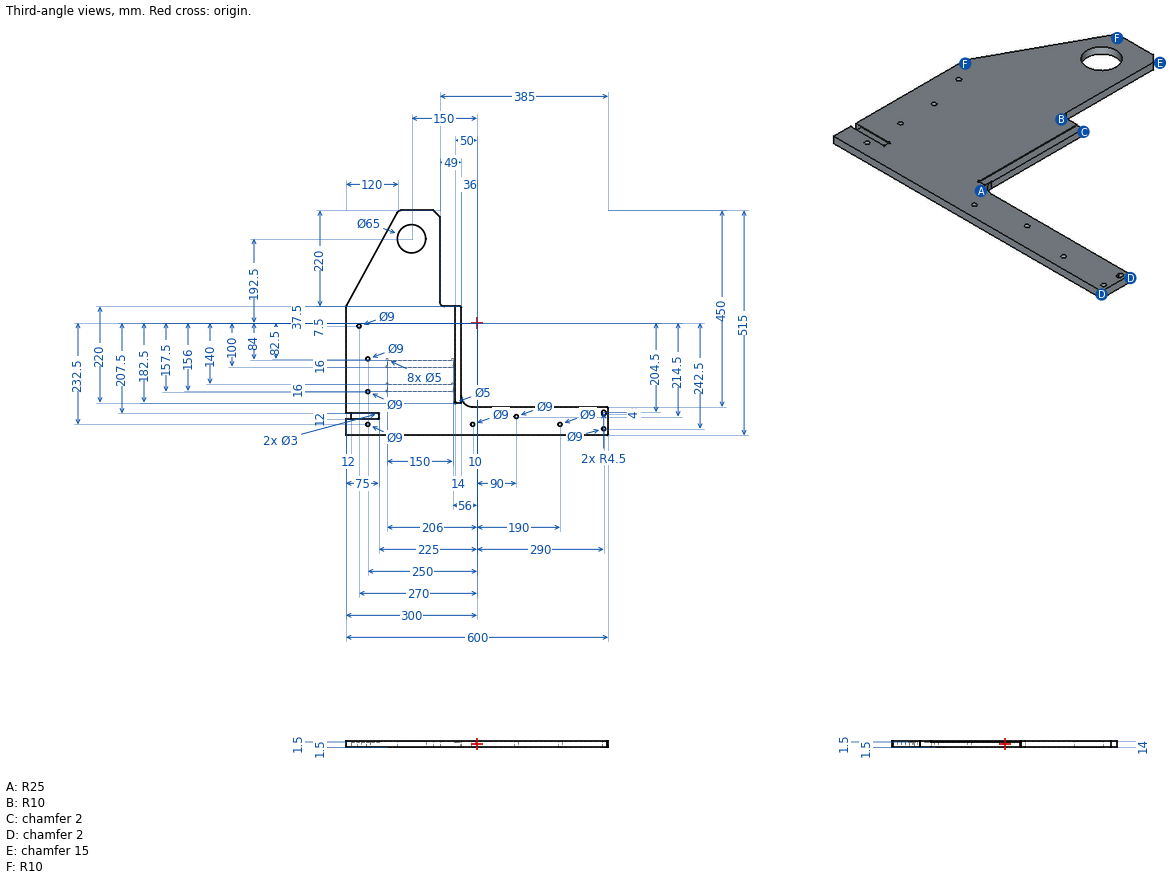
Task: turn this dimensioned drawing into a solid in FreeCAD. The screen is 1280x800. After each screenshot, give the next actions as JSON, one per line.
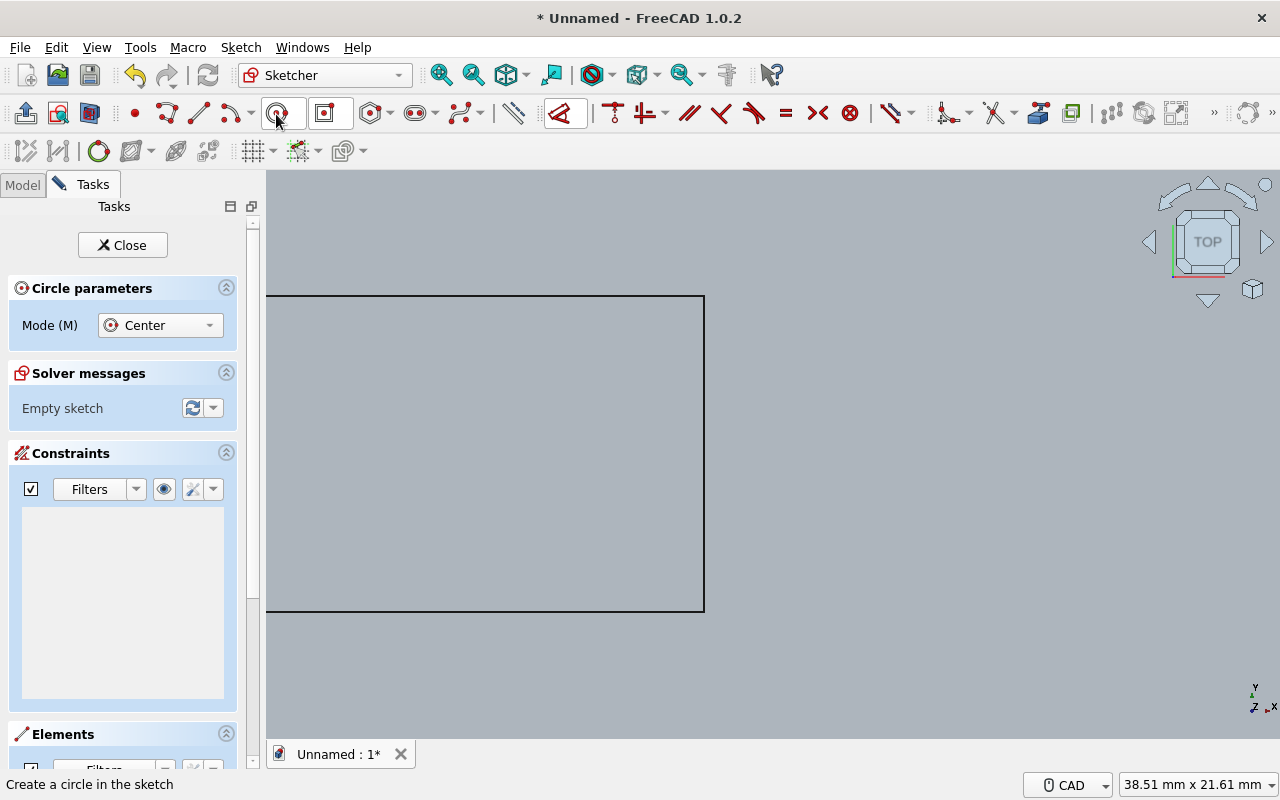
{"action": "left_click", "coordinate": [704, 296]}
{"action": "mouse_move", "coordinate": [732, 268]}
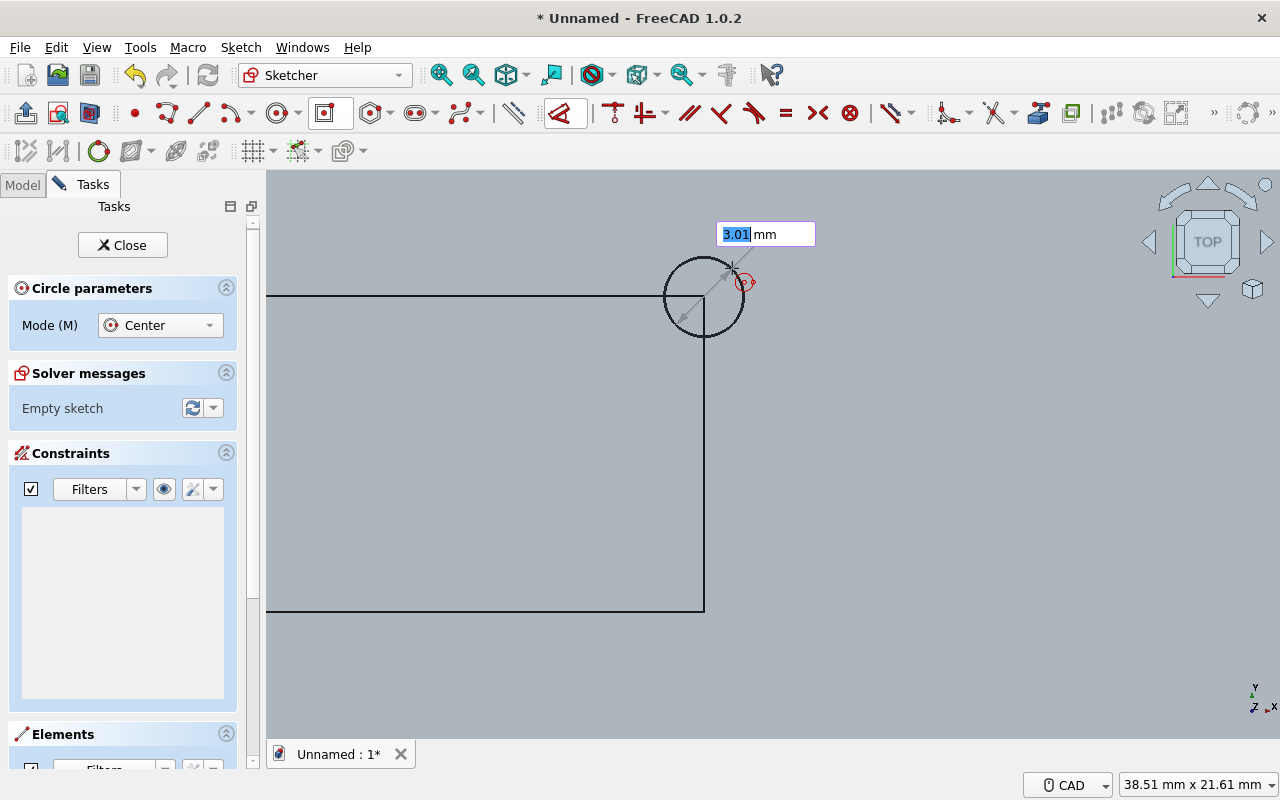
{"action": "type", "text": "3"}
{"action": "key", "text": "Return"}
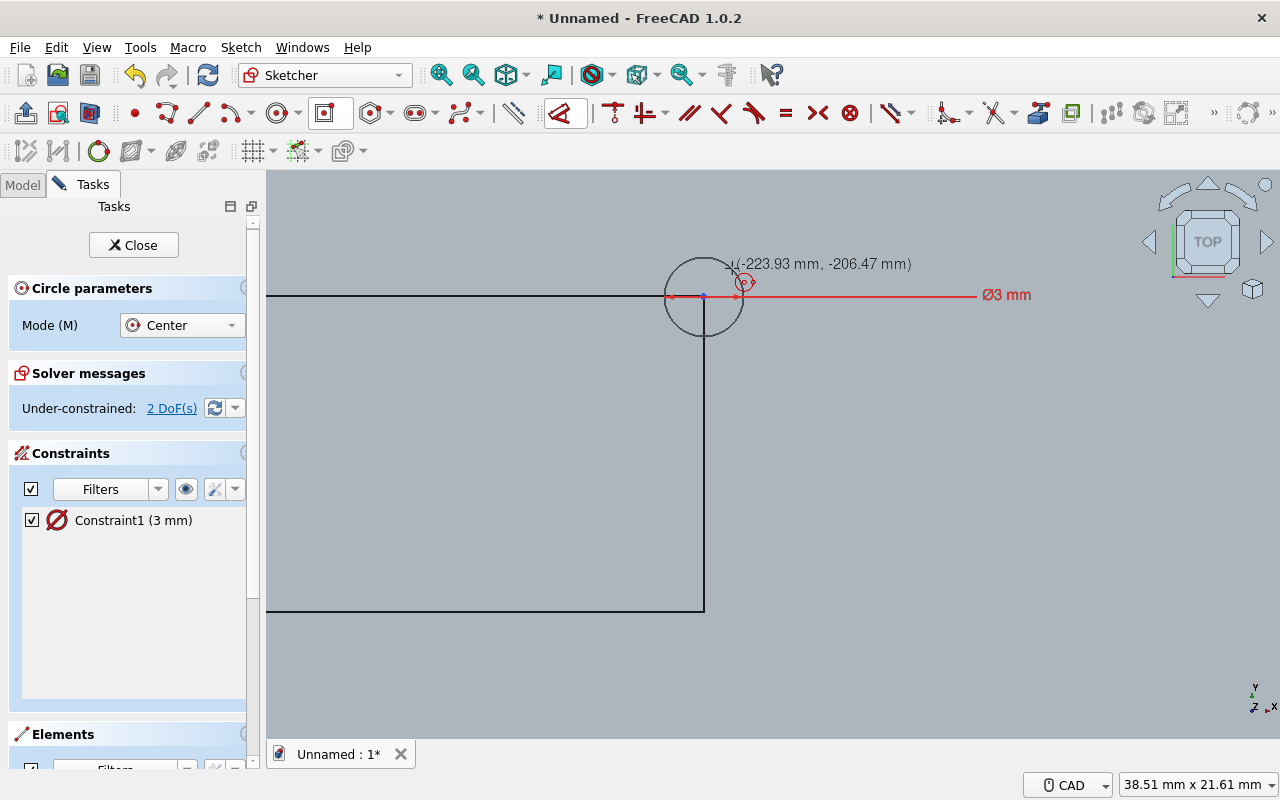
{"action": "left_click", "coordinate": [704, 612]}
{"action": "mouse_move", "coordinate": [732, 584]}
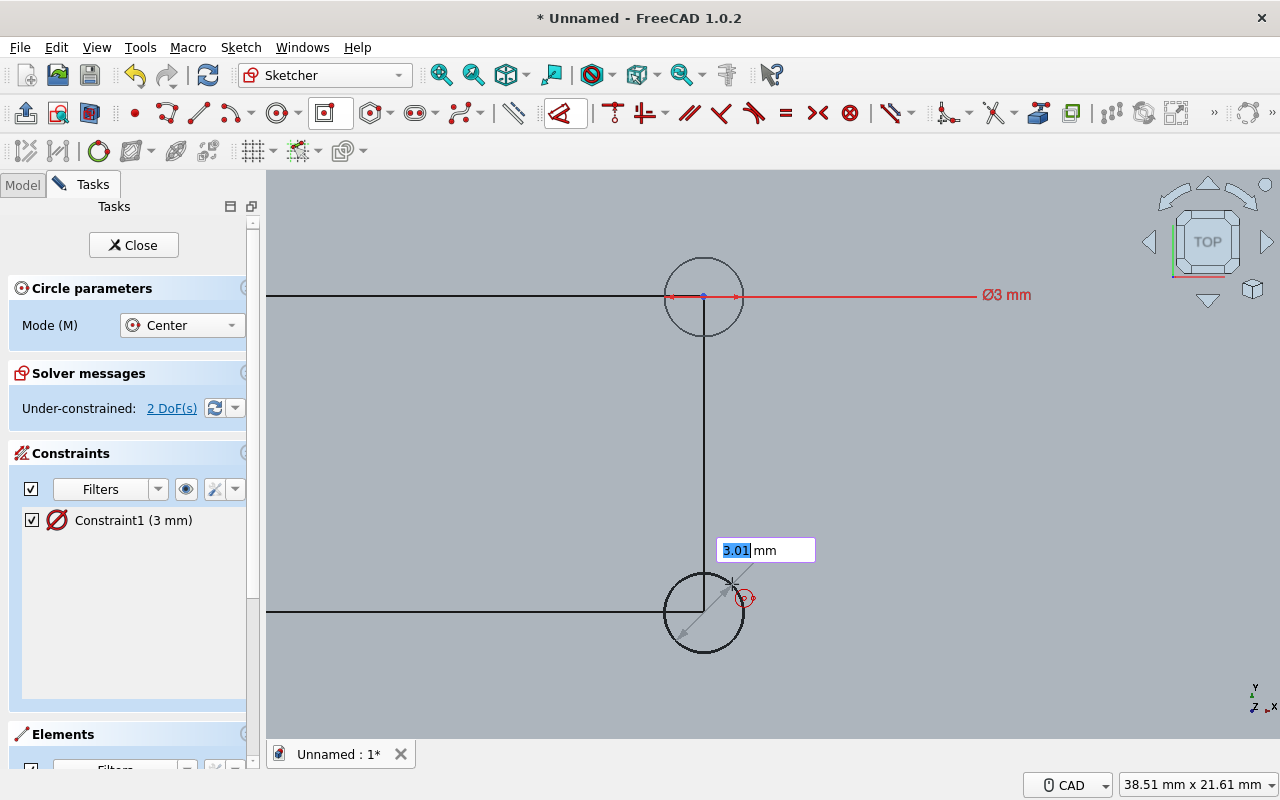
{"action": "type", "text": "3"}
{"action": "key", "text": "Return"}
{"action": "key", "text": "Escape"}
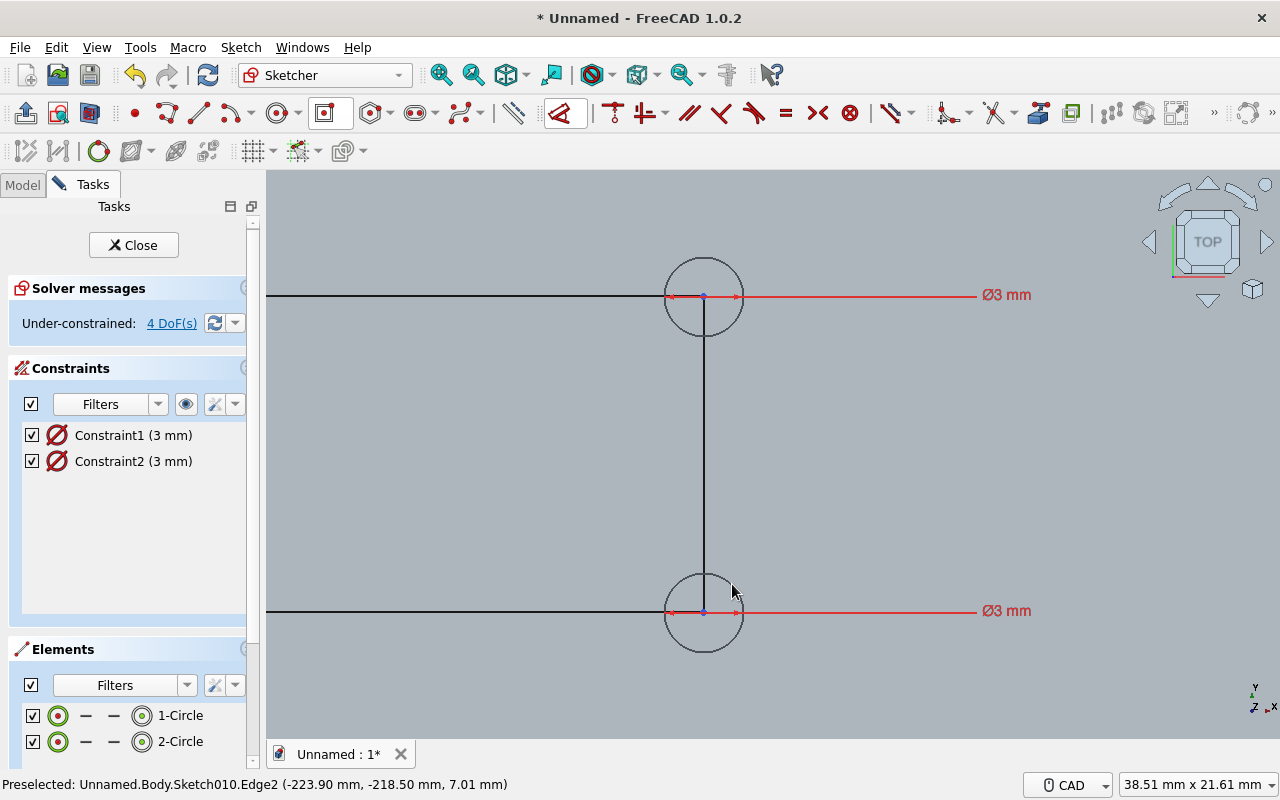
{"action": "left_click", "coordinate": [704, 297]}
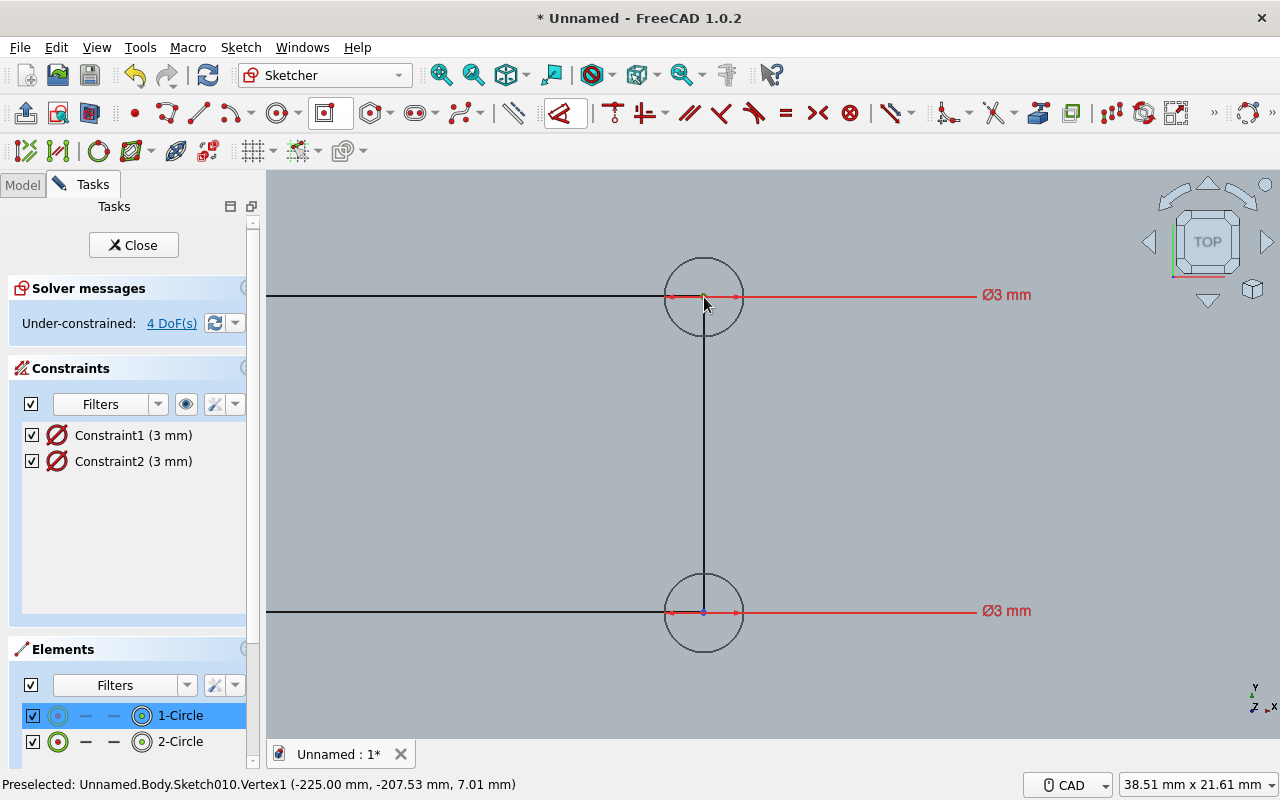
{"action": "key", "text": "l"}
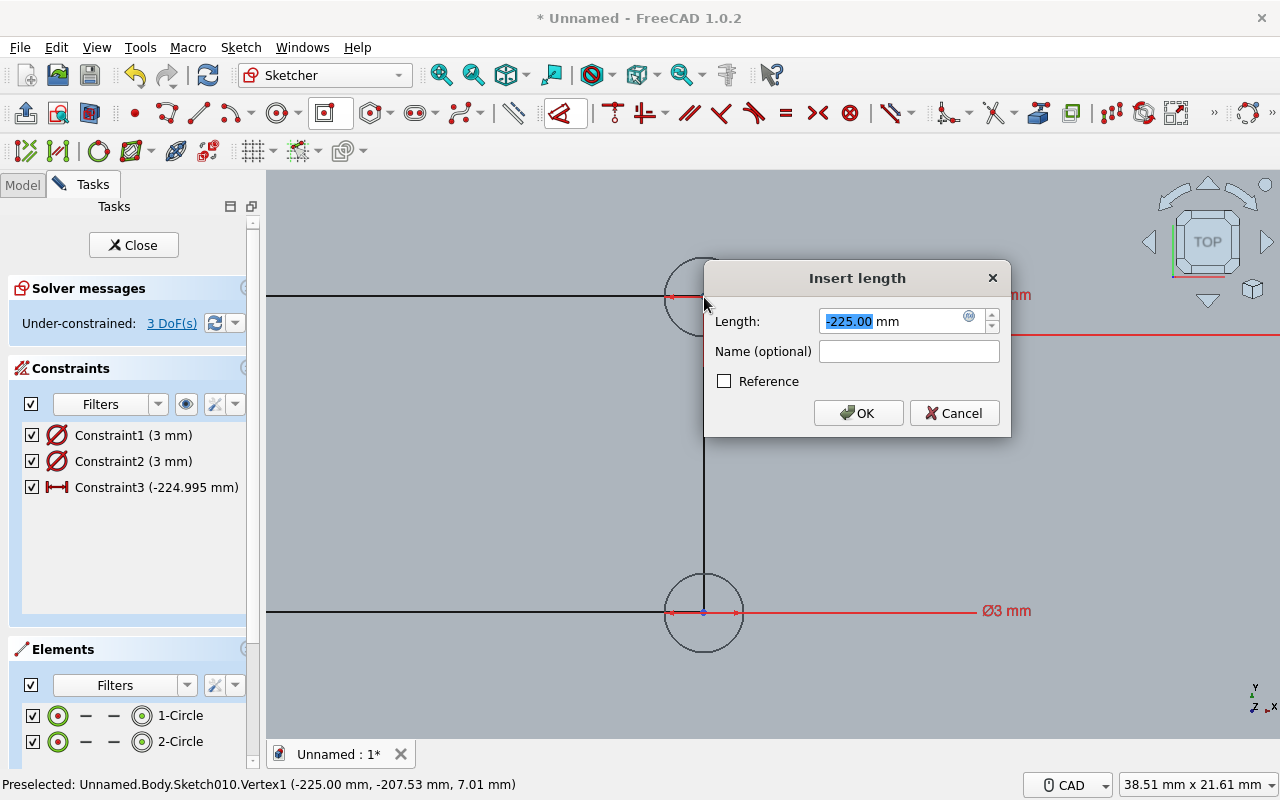
{"action": "type", "text": "-225"}
{"action": "key", "text": "Return"}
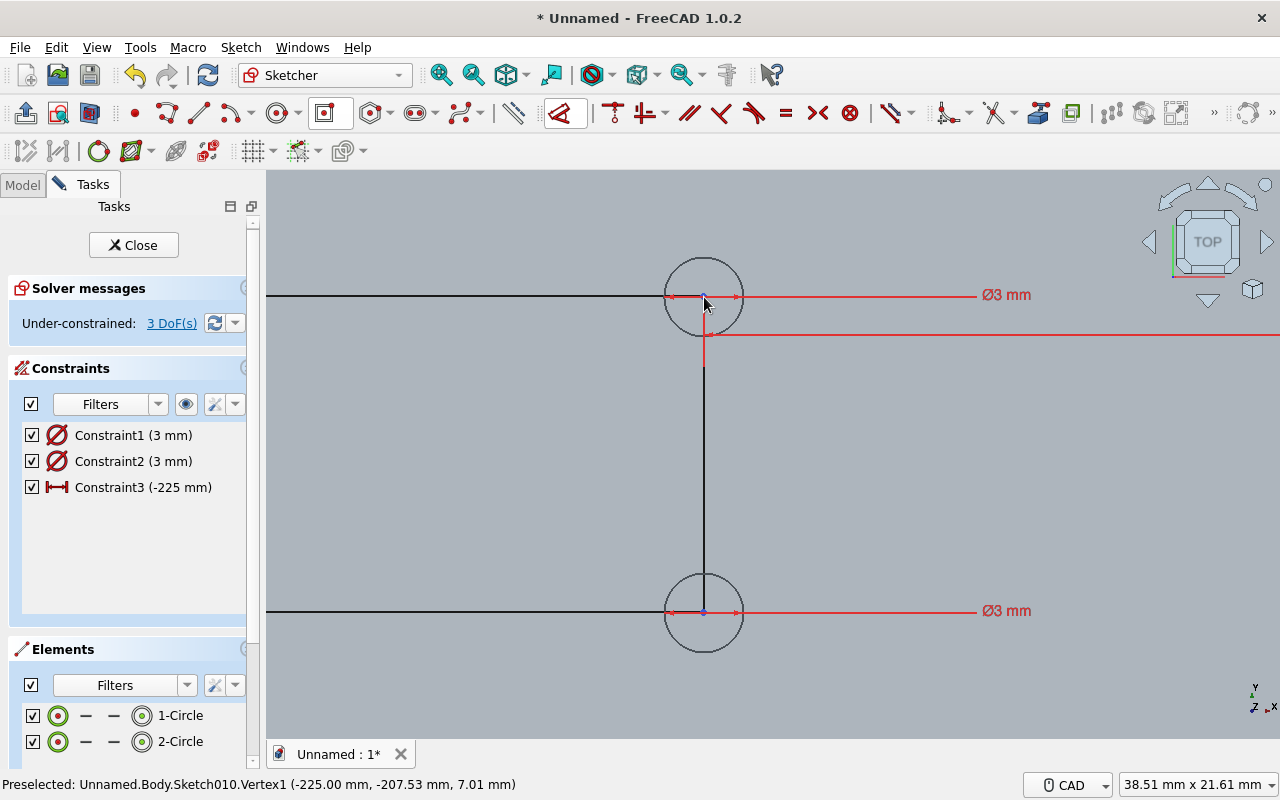
{"action": "left_click", "coordinate": [704, 613]}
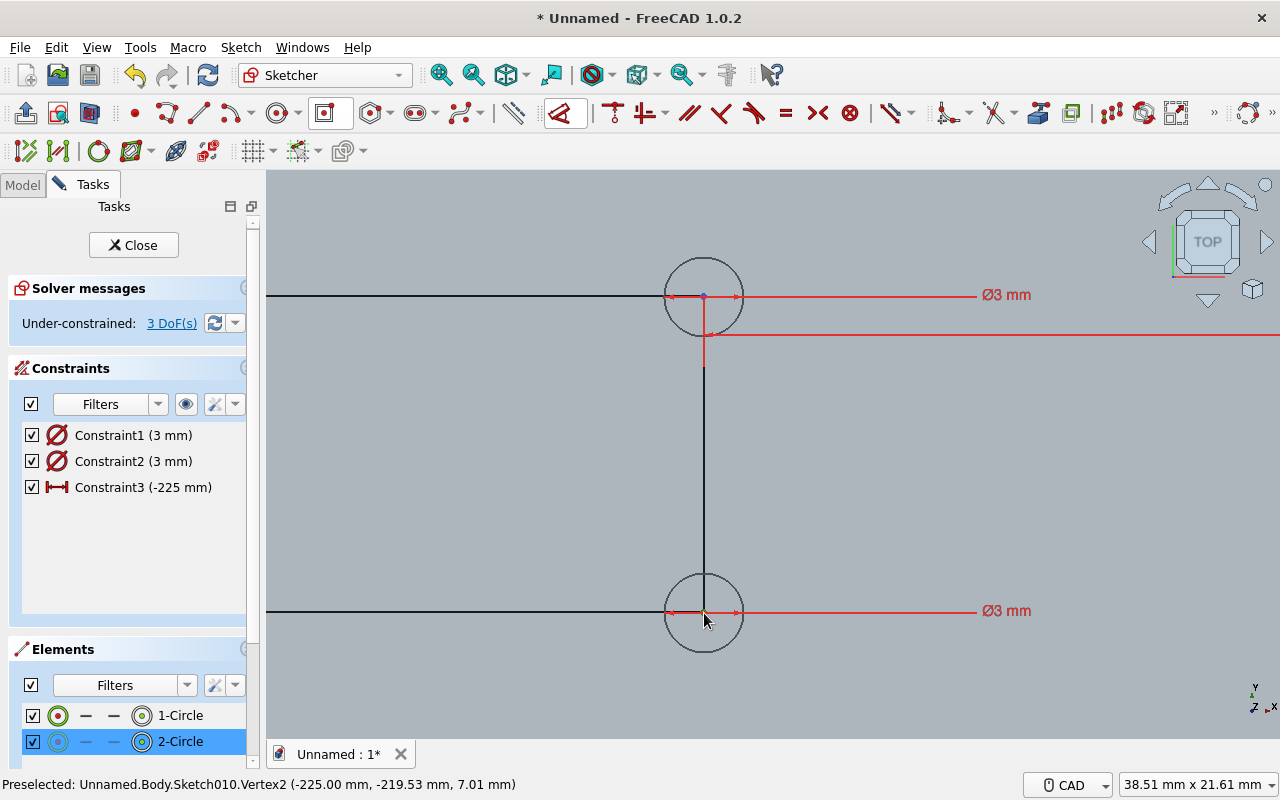
{"action": "left_click", "coordinate": [582, 114]}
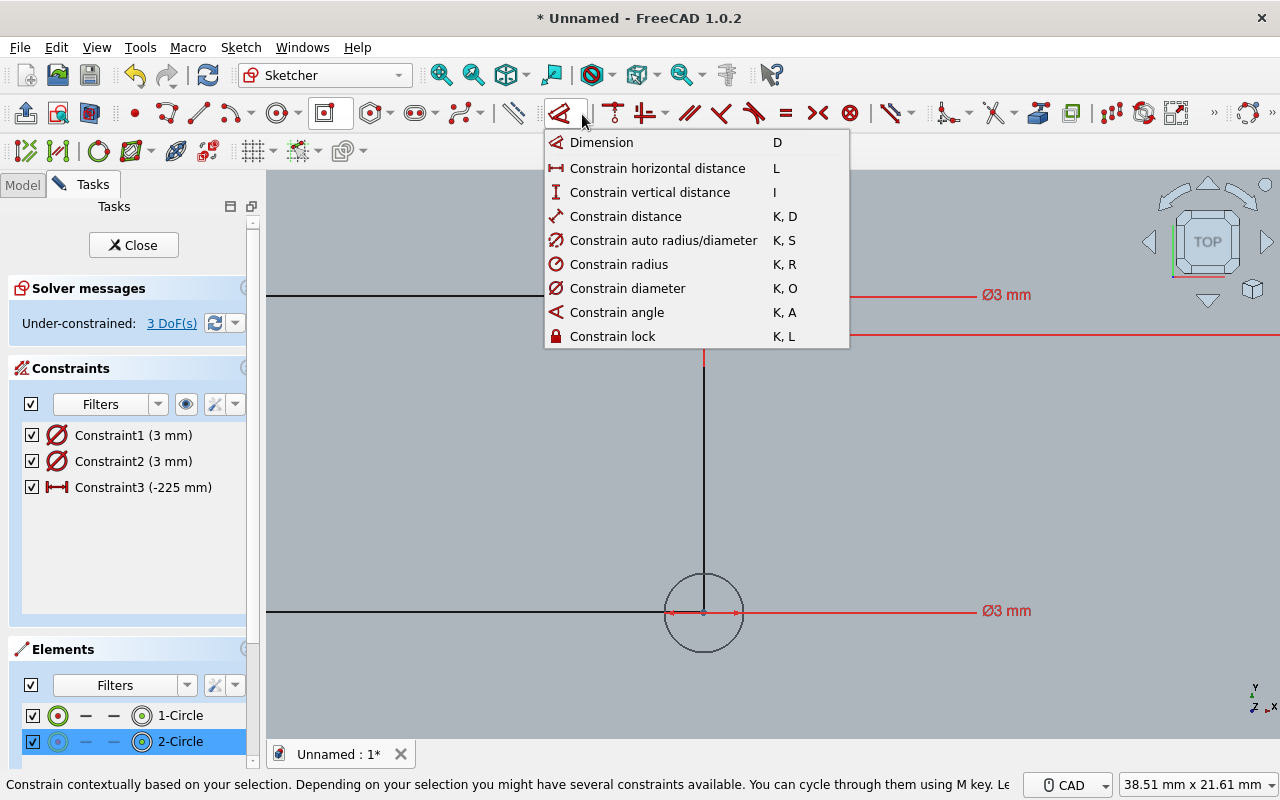
{"action": "left_click", "coordinate": [697, 168]}